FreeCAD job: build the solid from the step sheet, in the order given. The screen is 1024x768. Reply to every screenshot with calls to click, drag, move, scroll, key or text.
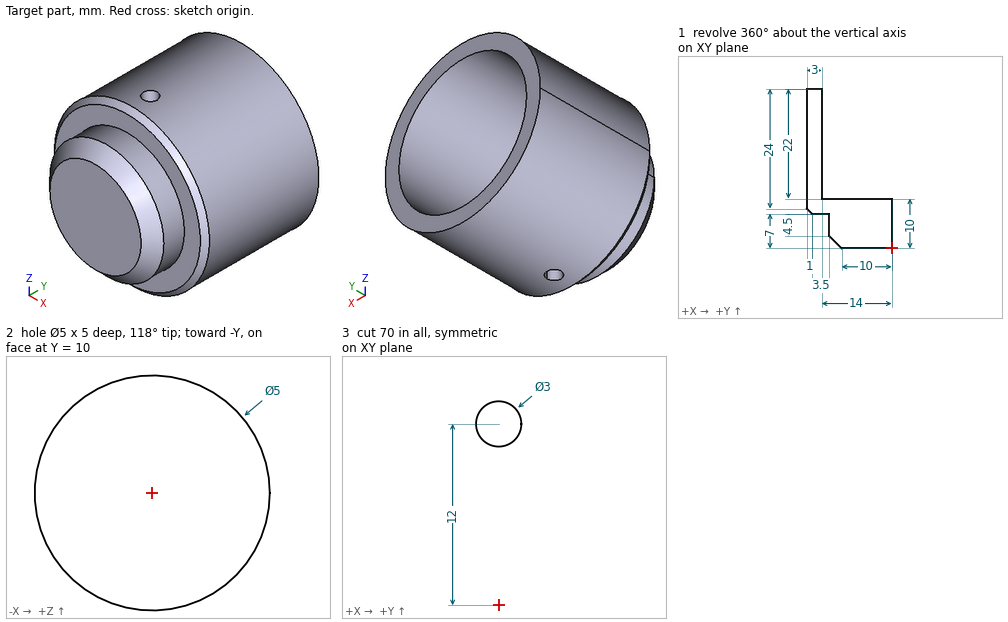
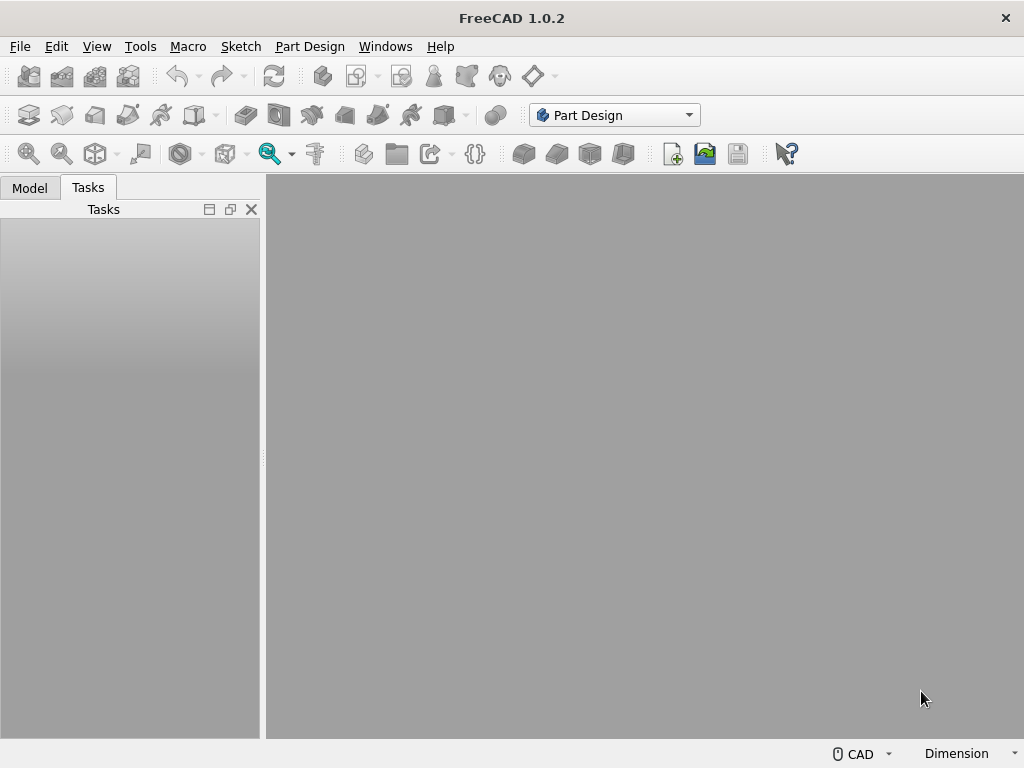
key(ctrl+n)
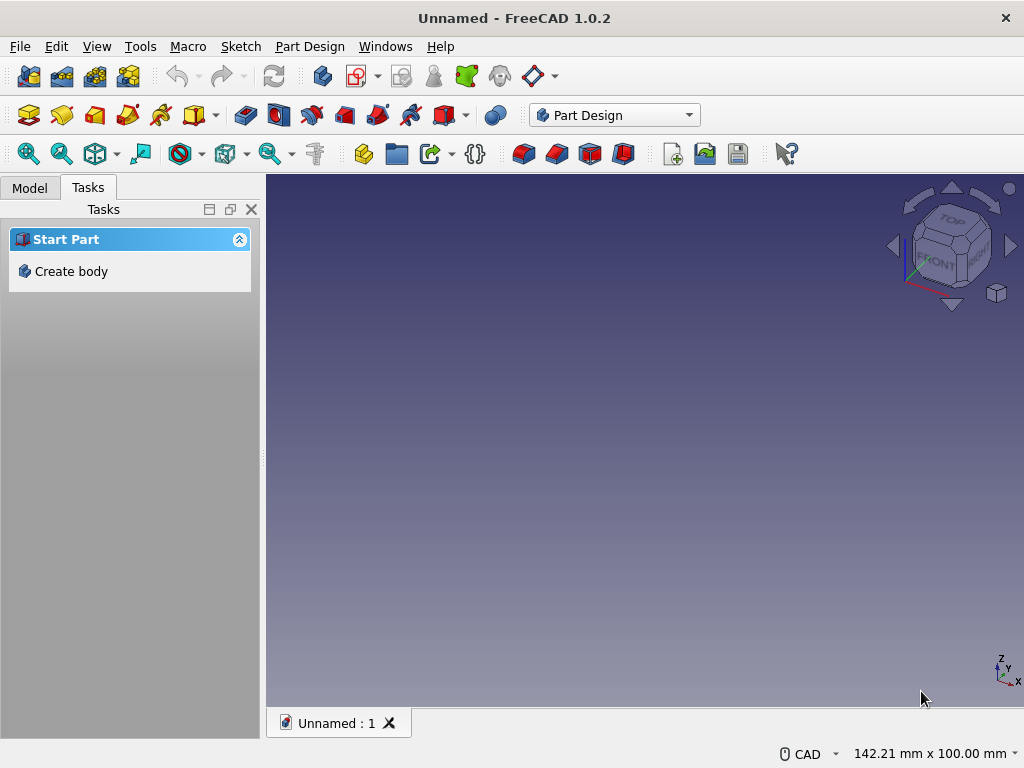
click(356, 76)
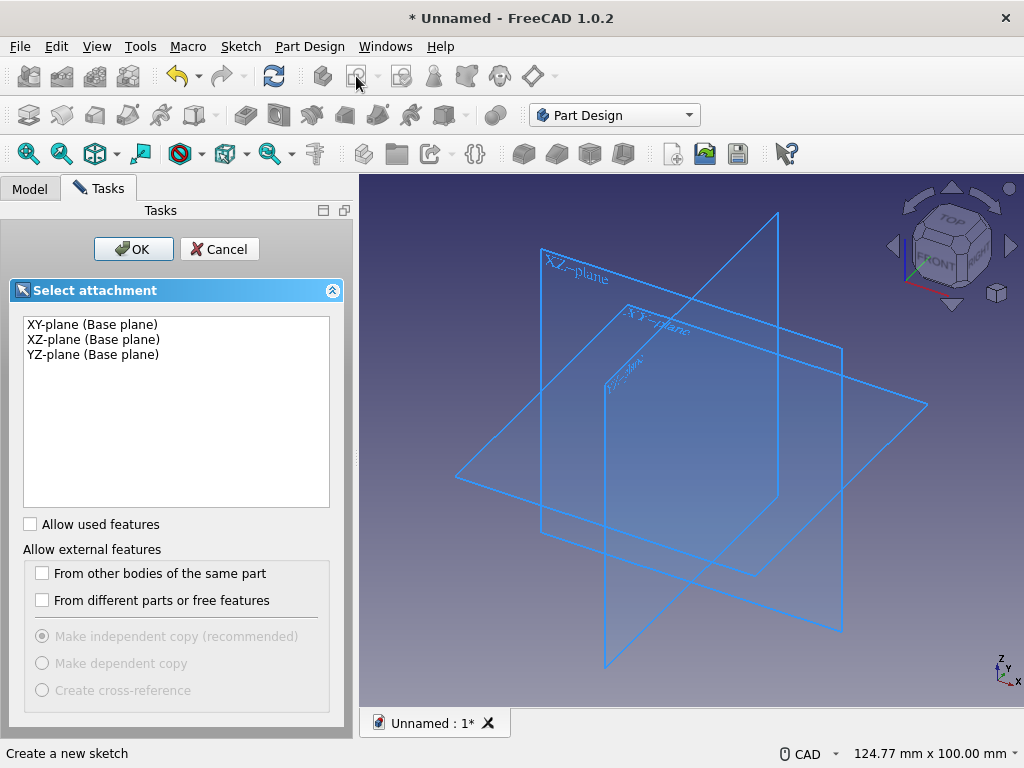
click(84, 324)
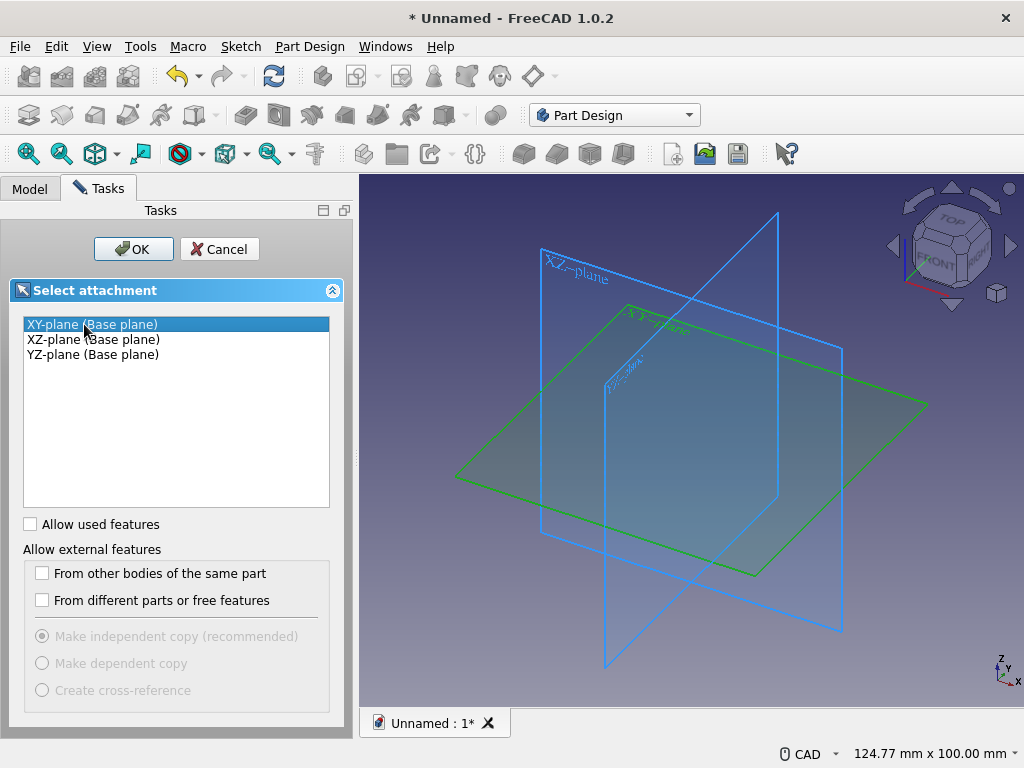
click(134, 249)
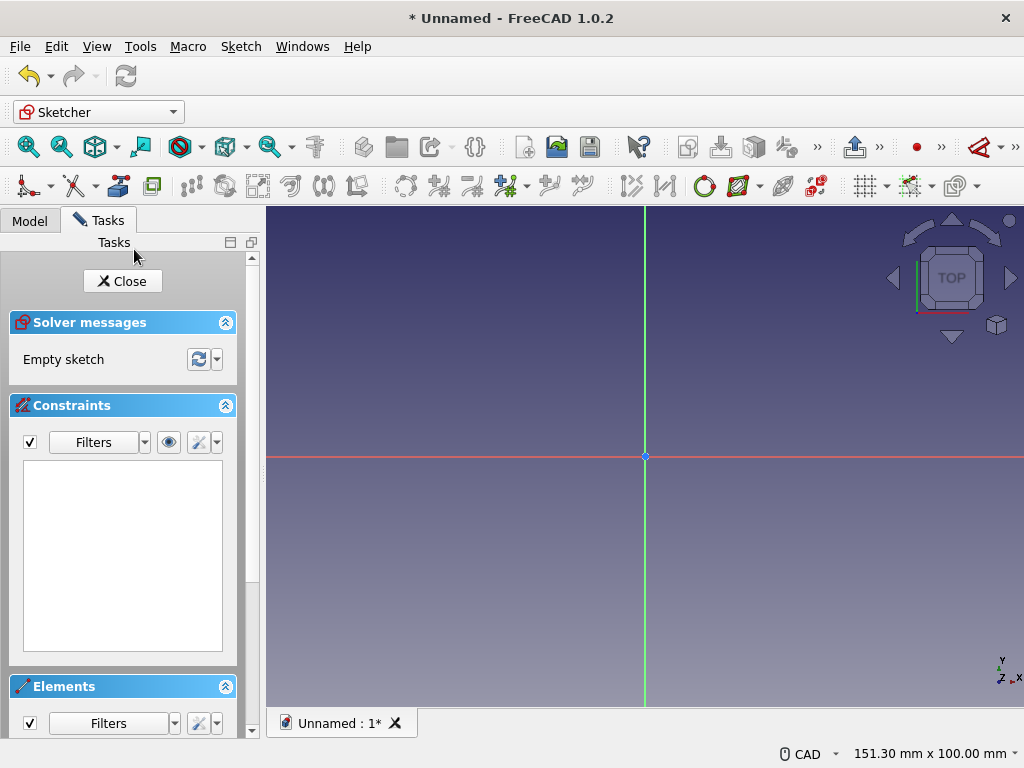
scroll(634, 279, up, 3)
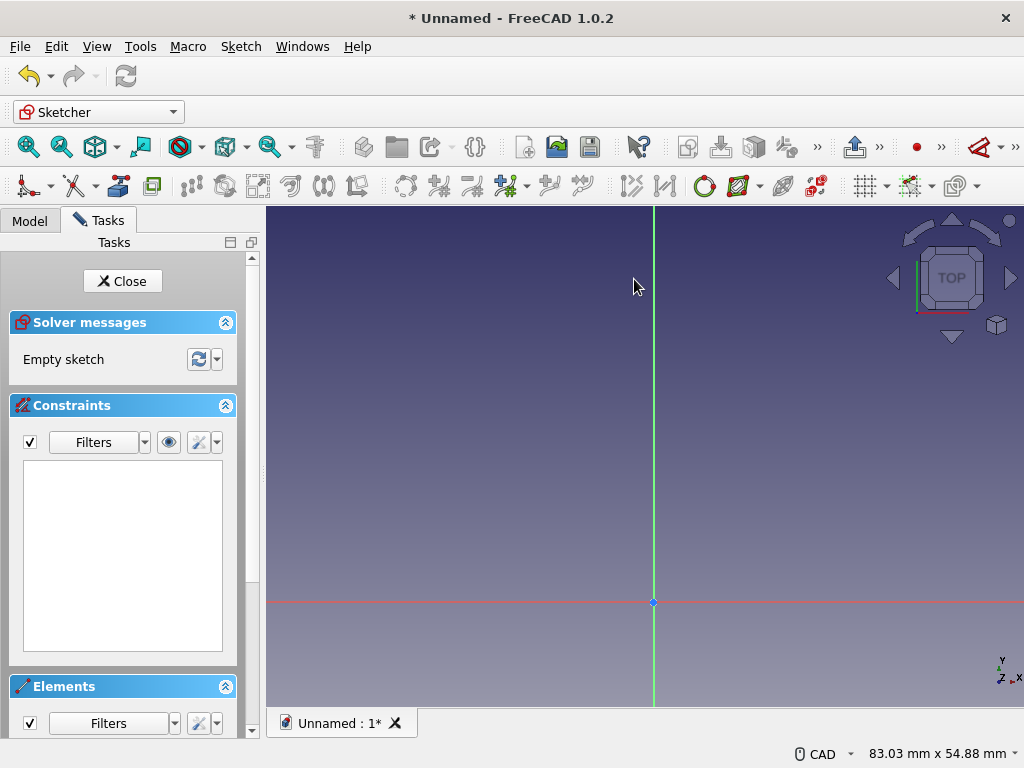
key(g)
key(m)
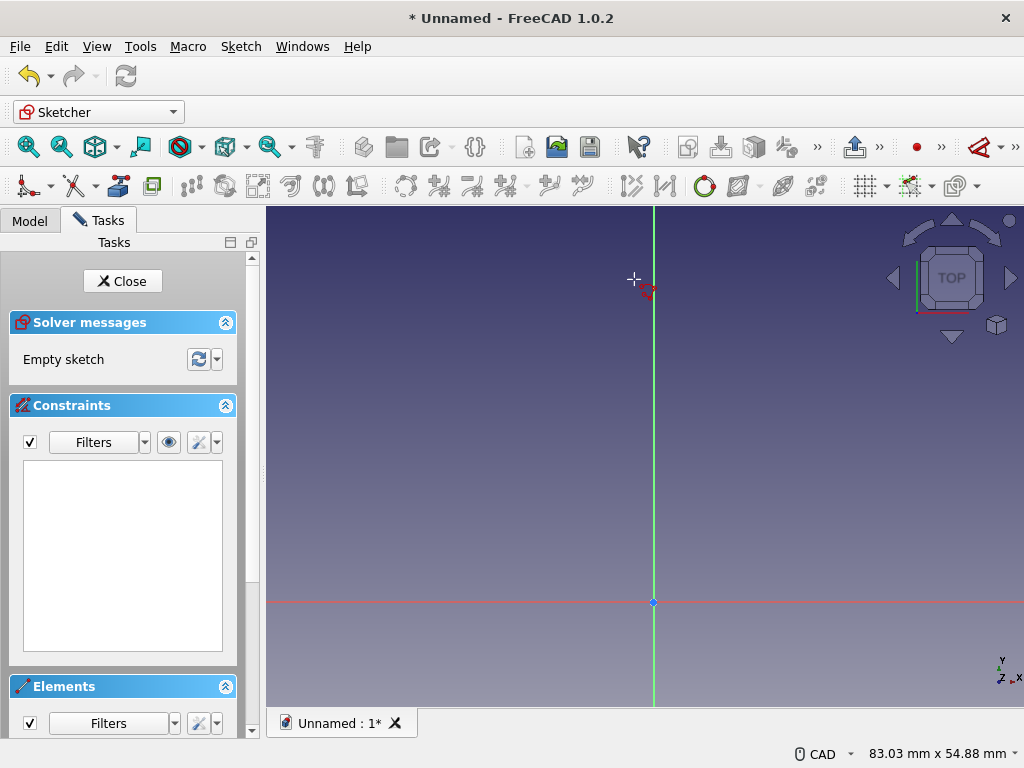
click(654, 602)
click(645, 511)
click(526, 511)
click(526, 310)
click(498, 310)
click(498, 529)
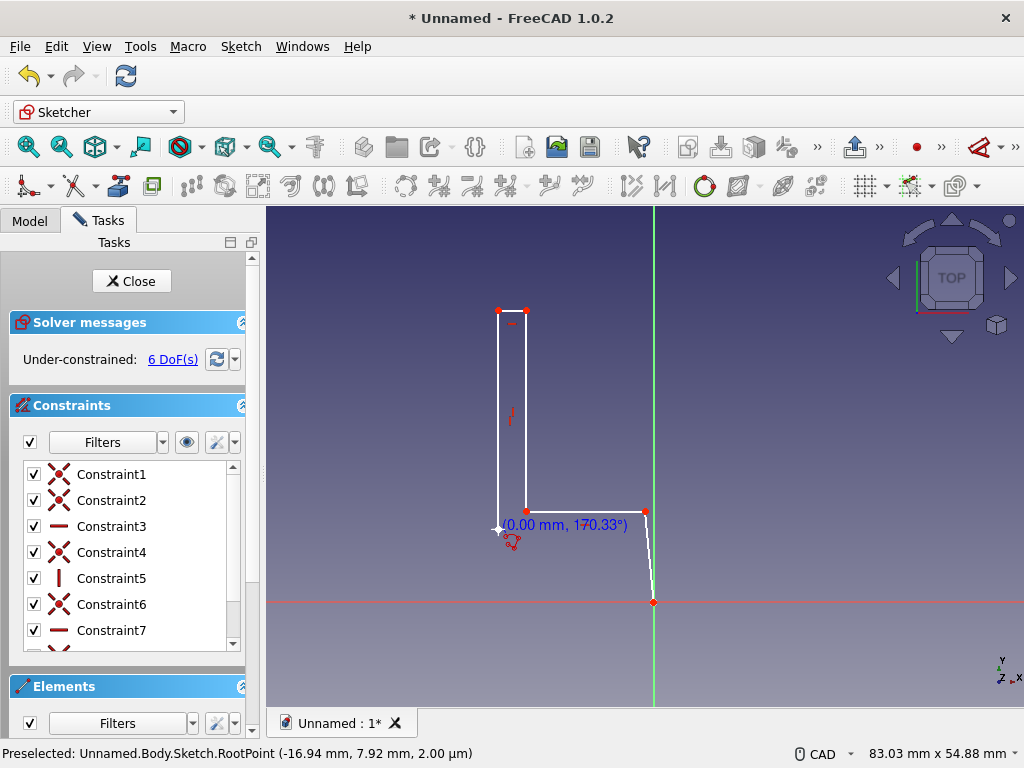
scroll(508, 538, up, 2)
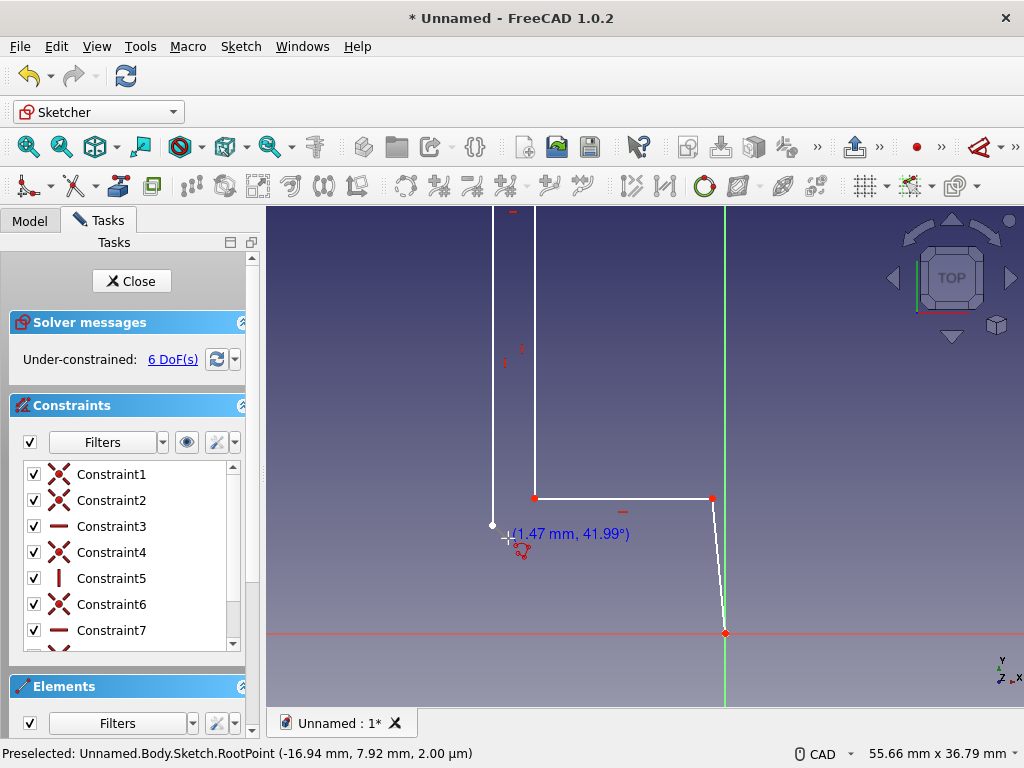
click(507, 538)
click(555, 538)
click(555, 600)
click(589, 625)
click(725, 634)
key(Escape)
key(Escape)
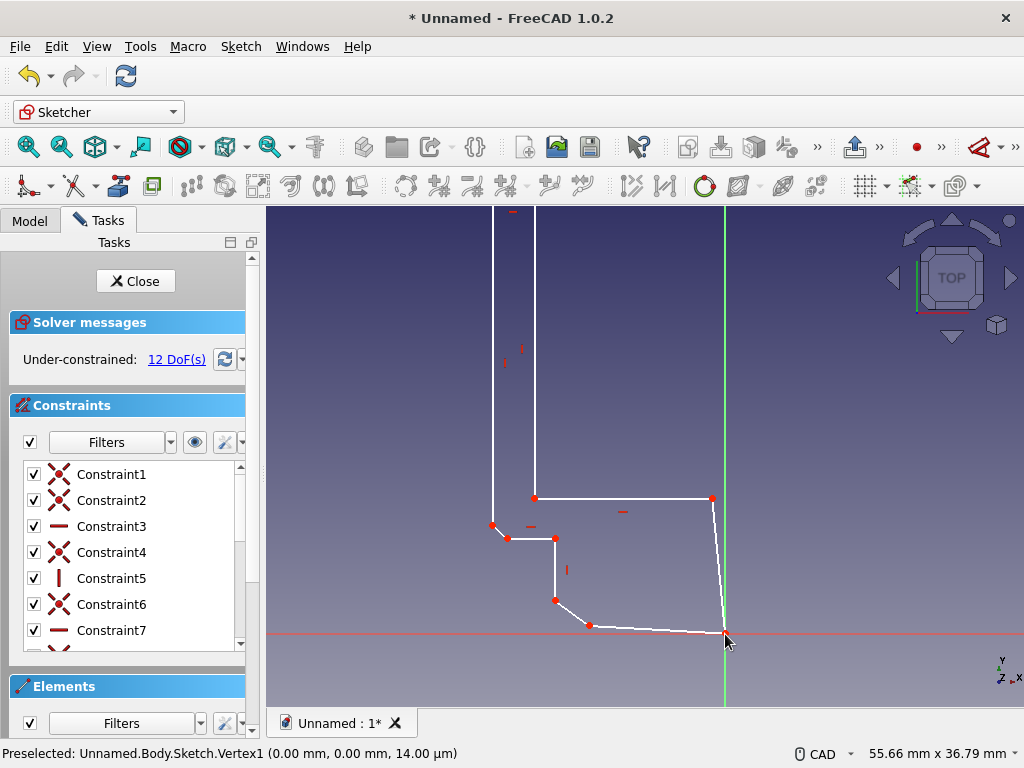
click(721, 593)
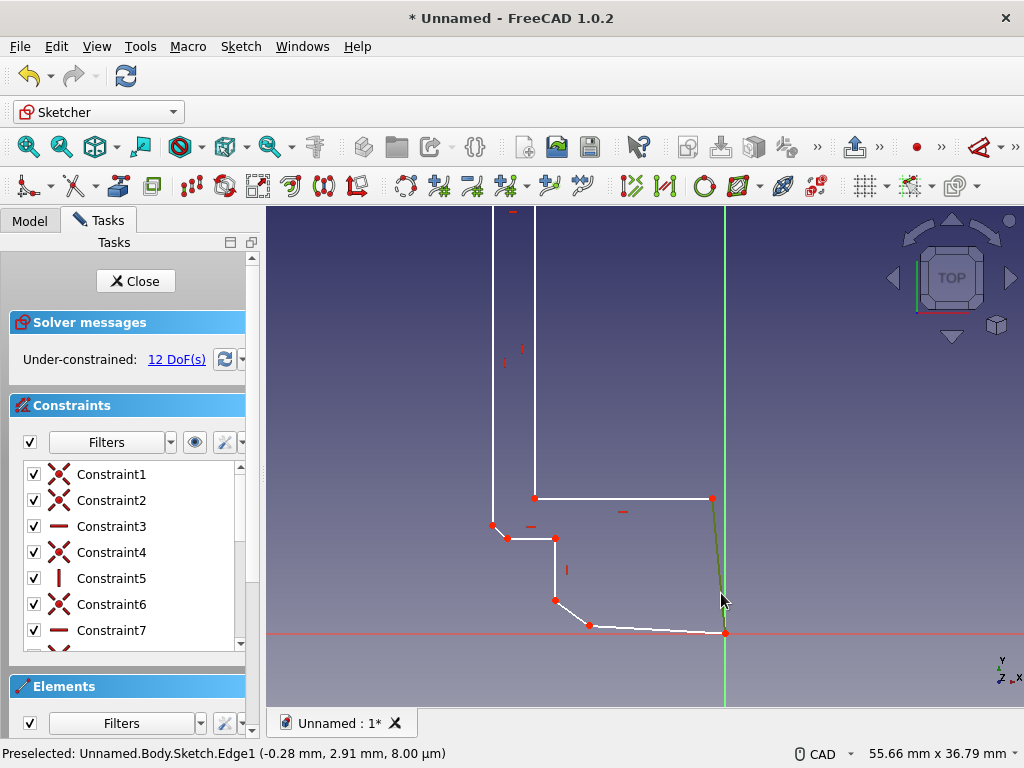
key(v)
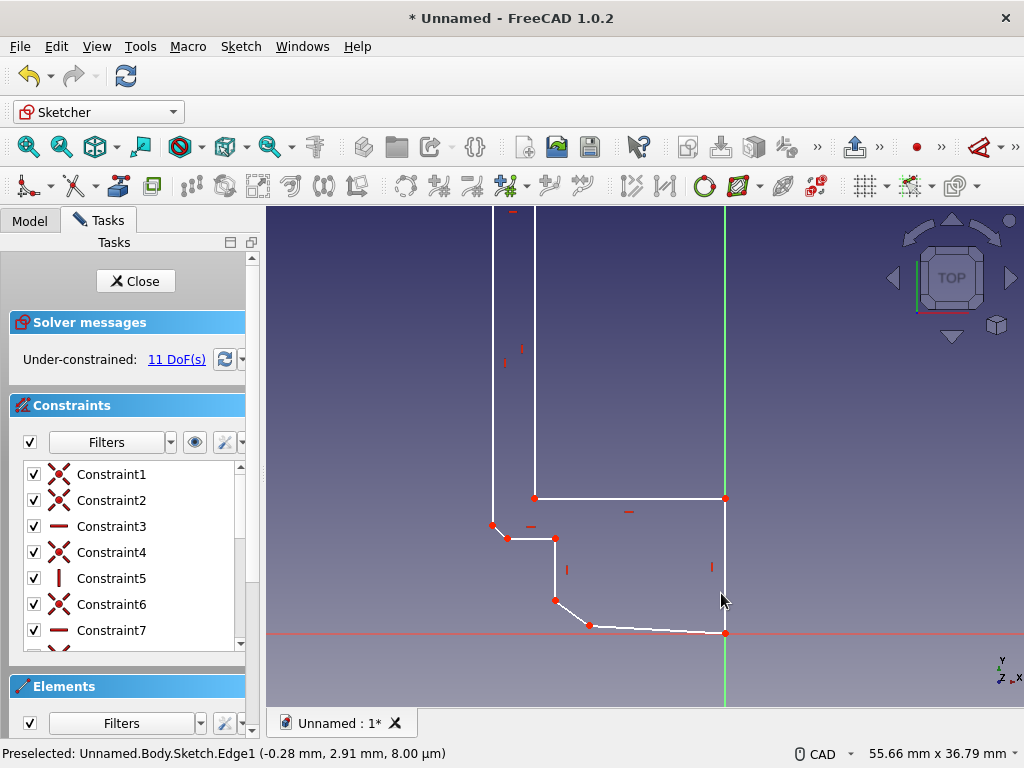
click(684, 631)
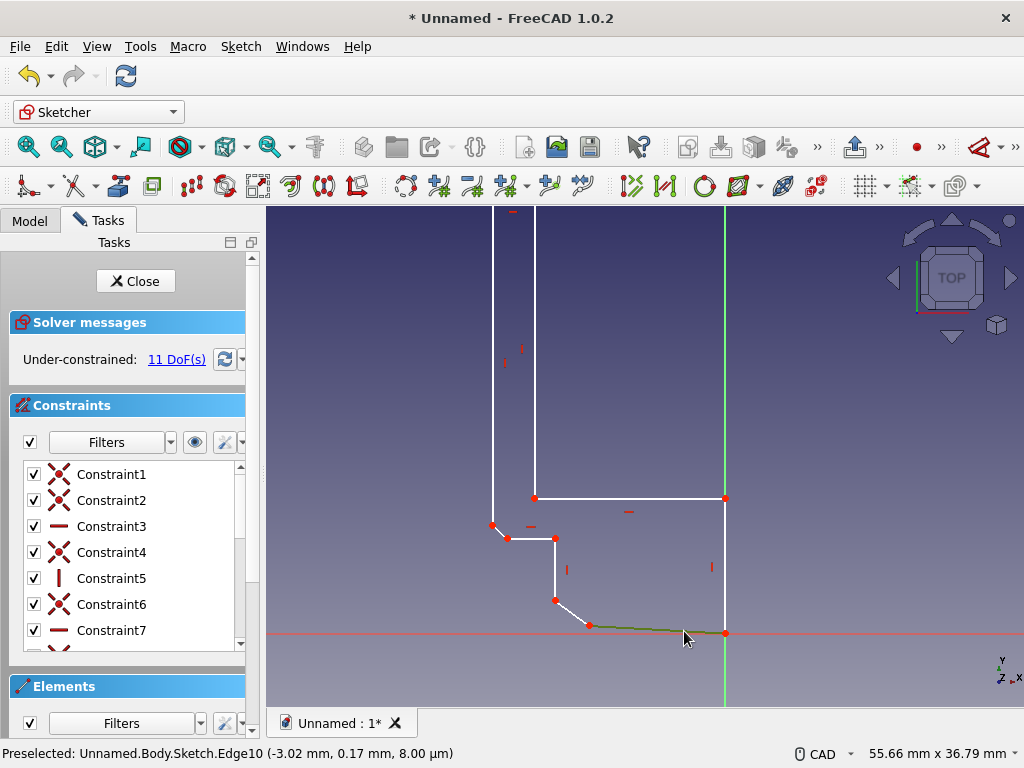
key(h)